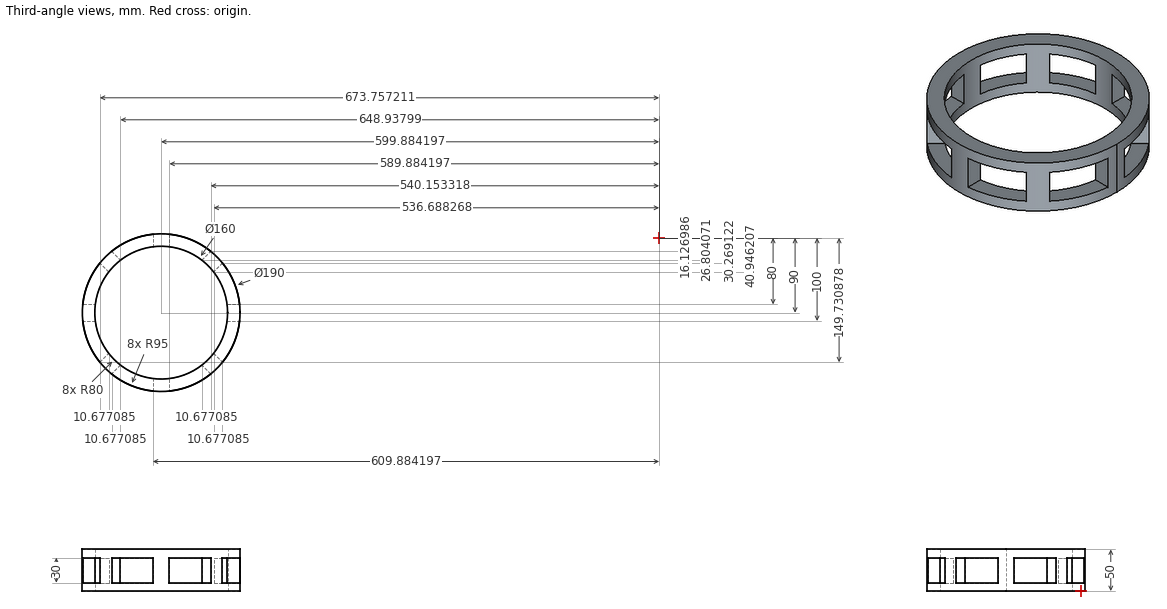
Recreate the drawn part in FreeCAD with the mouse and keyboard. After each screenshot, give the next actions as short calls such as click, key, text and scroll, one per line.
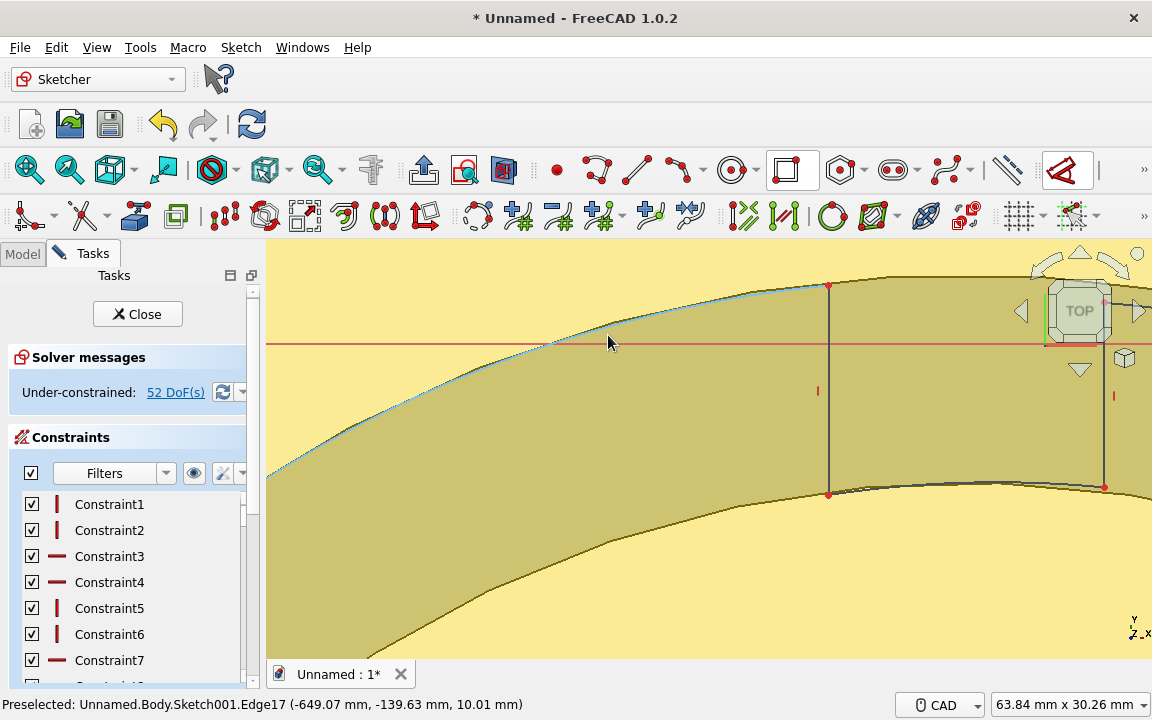
click(606, 327)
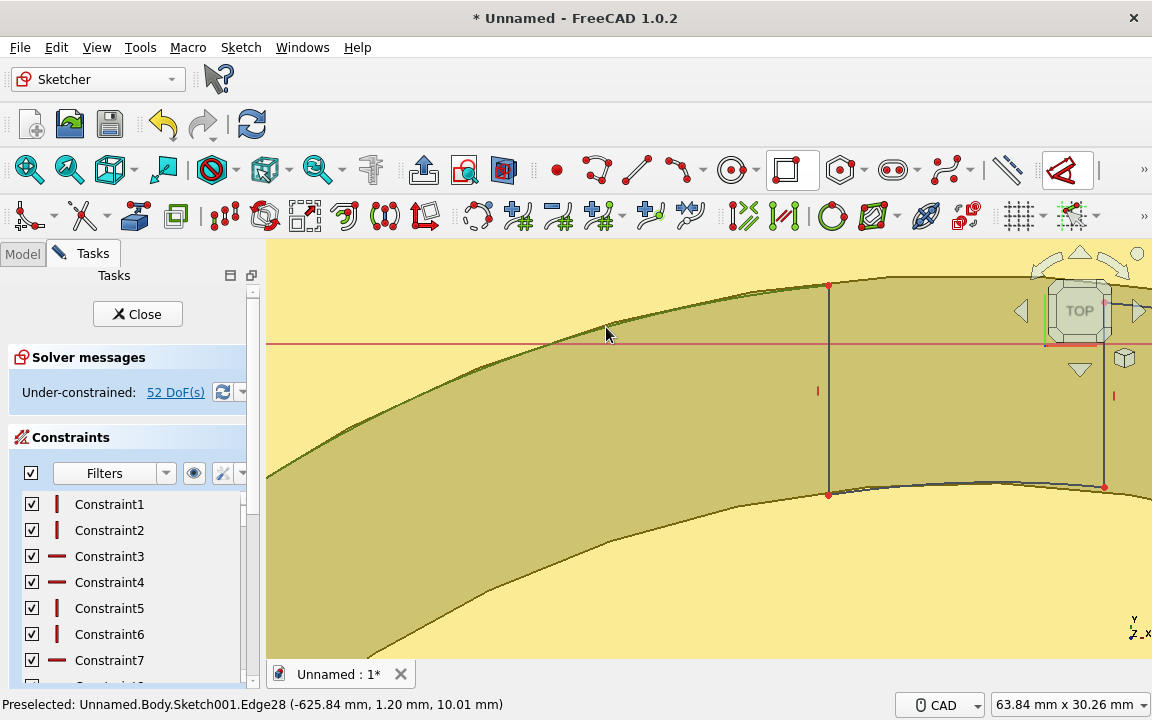
key(c)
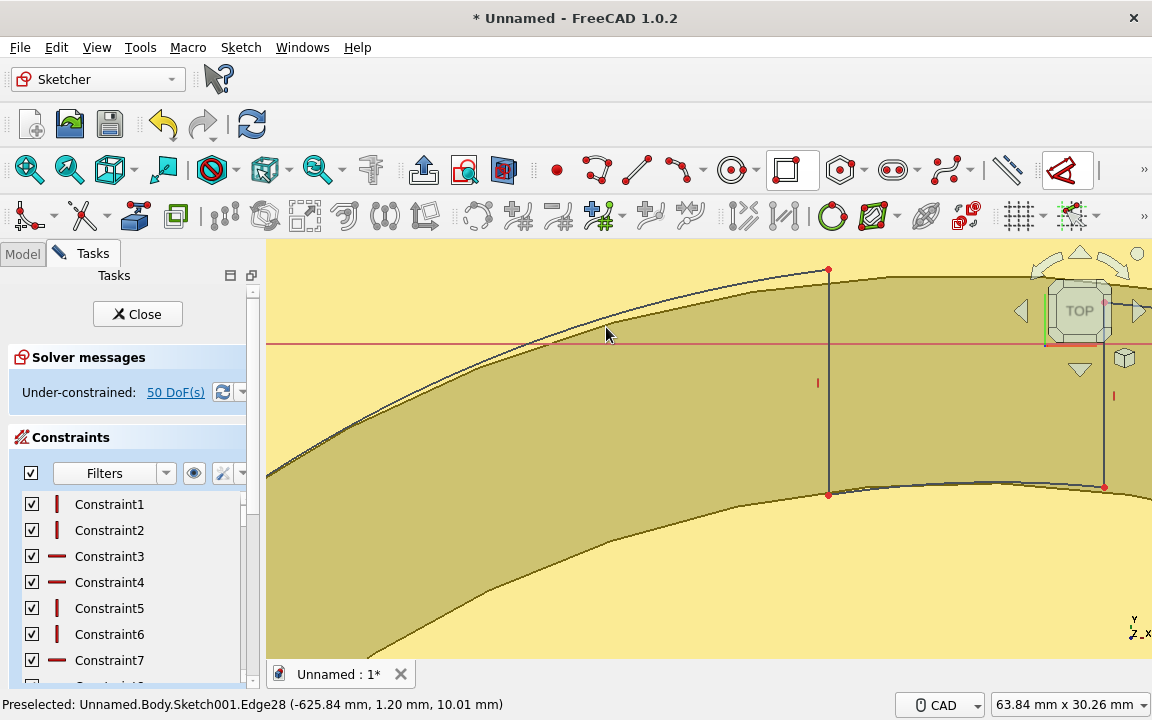
scroll(608, 335, down, 12)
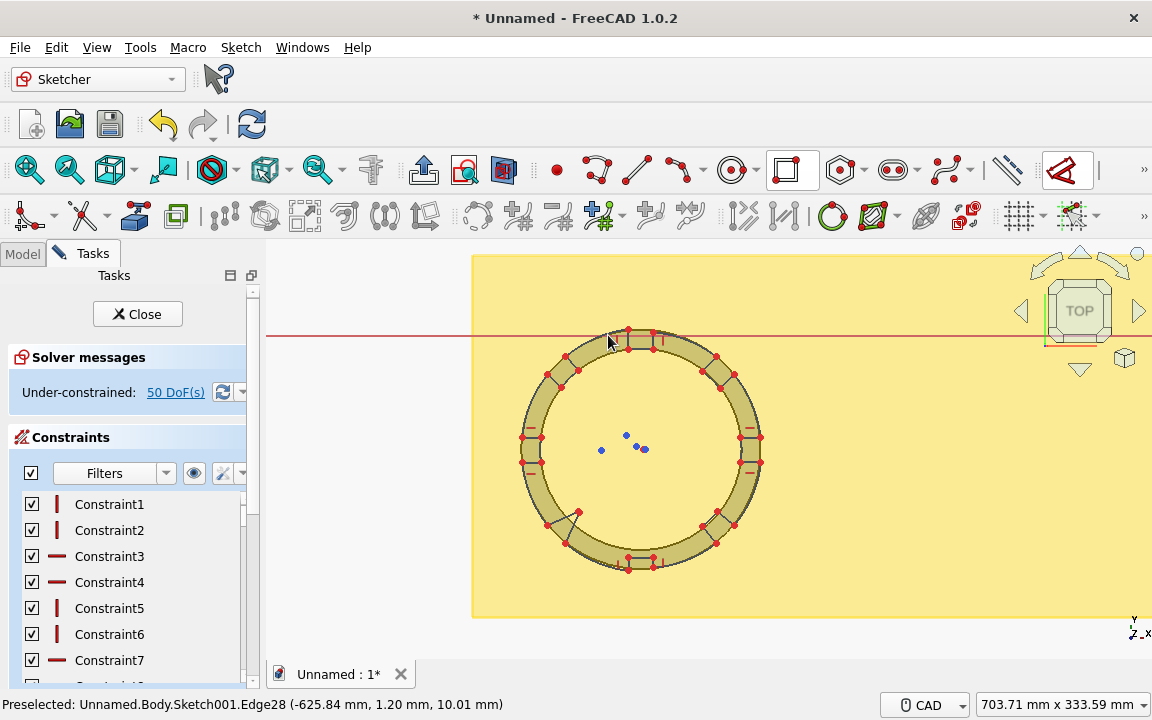
scroll(579, 512, up, 15)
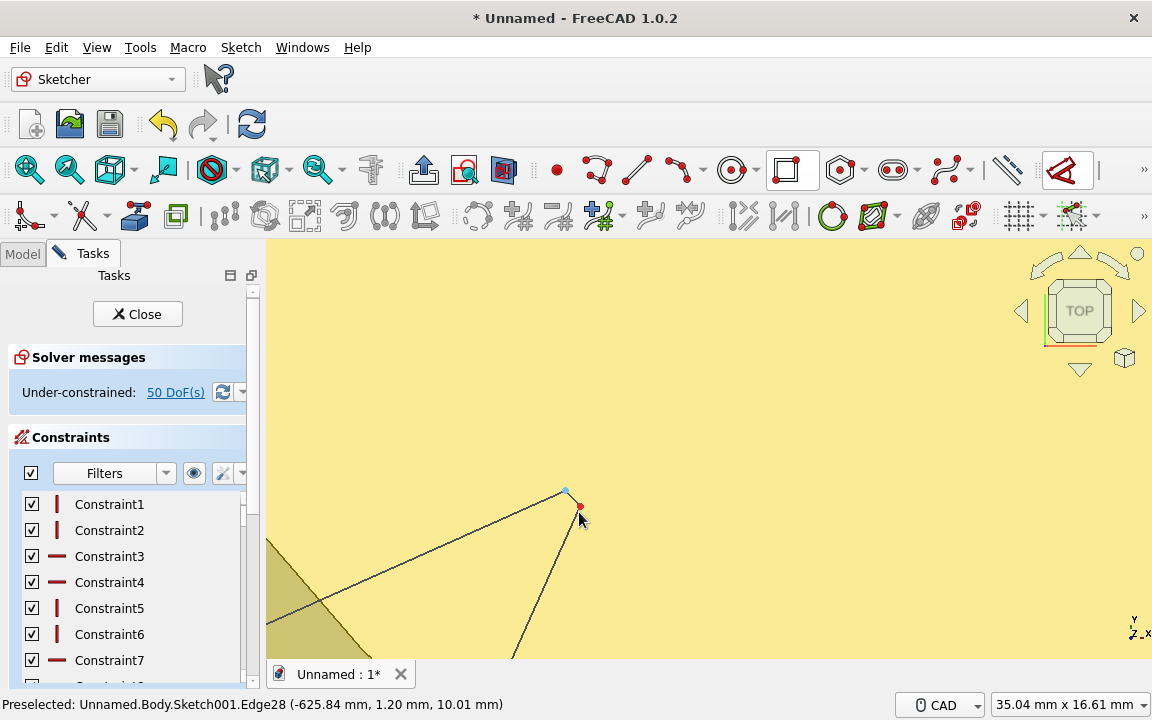
click(573, 499)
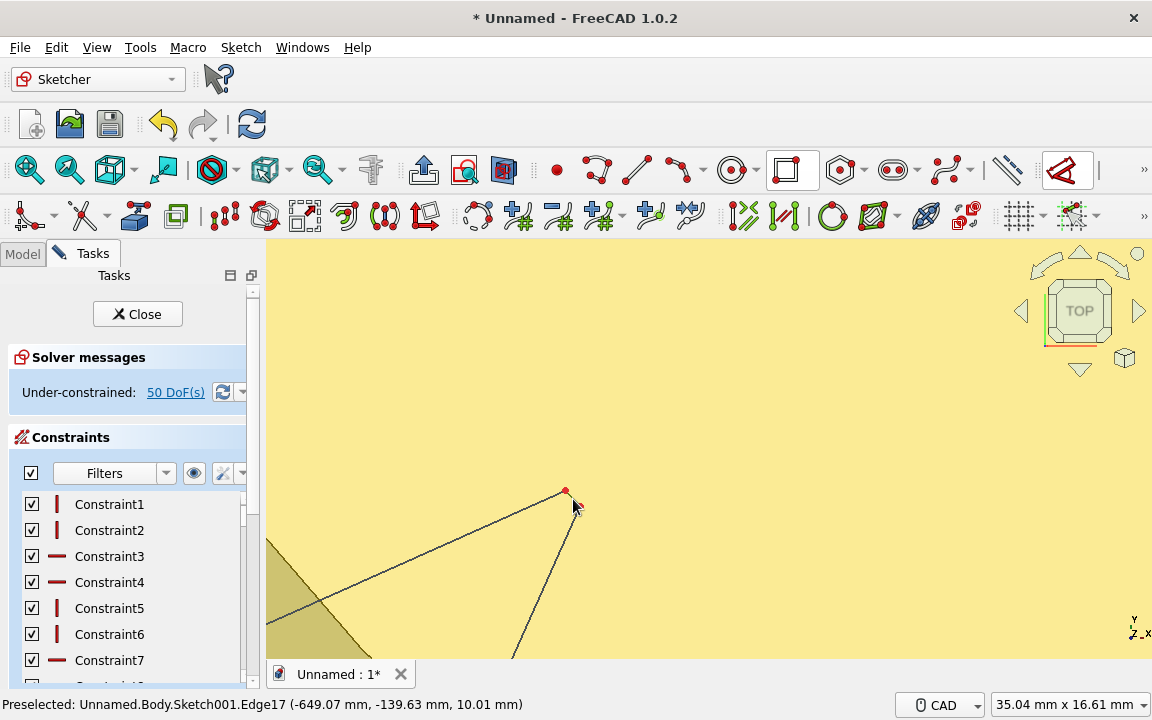
scroll(579, 512, down, 15)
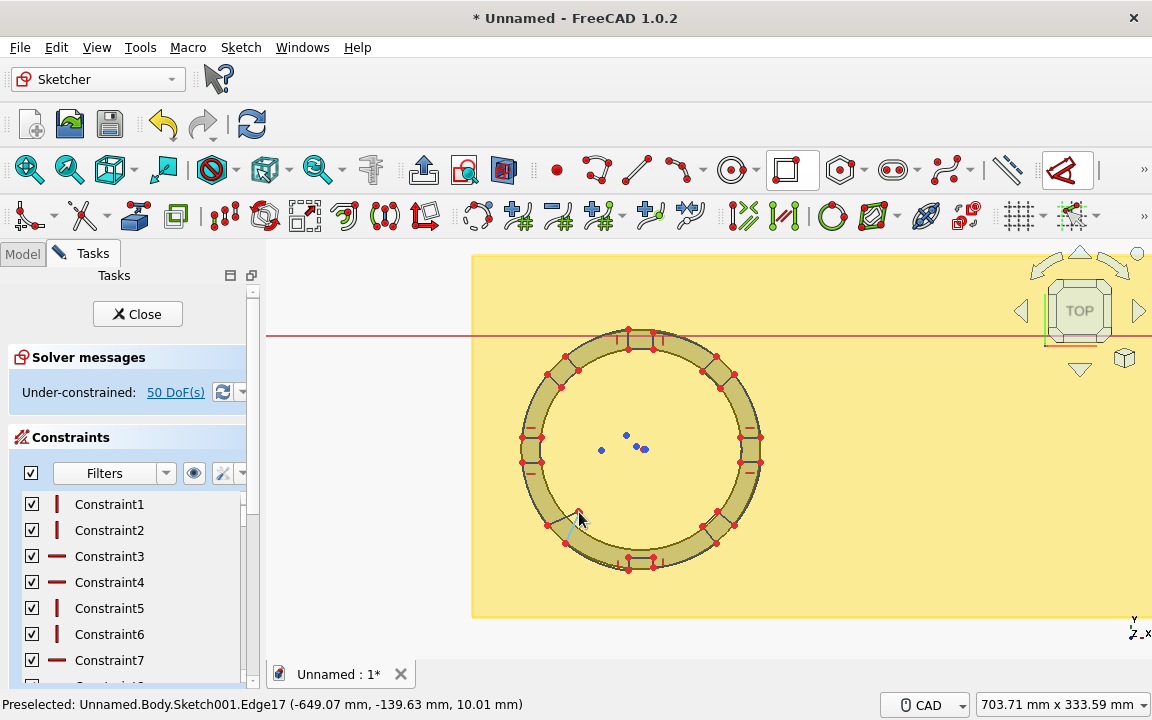
scroll(573, 375, up, 4)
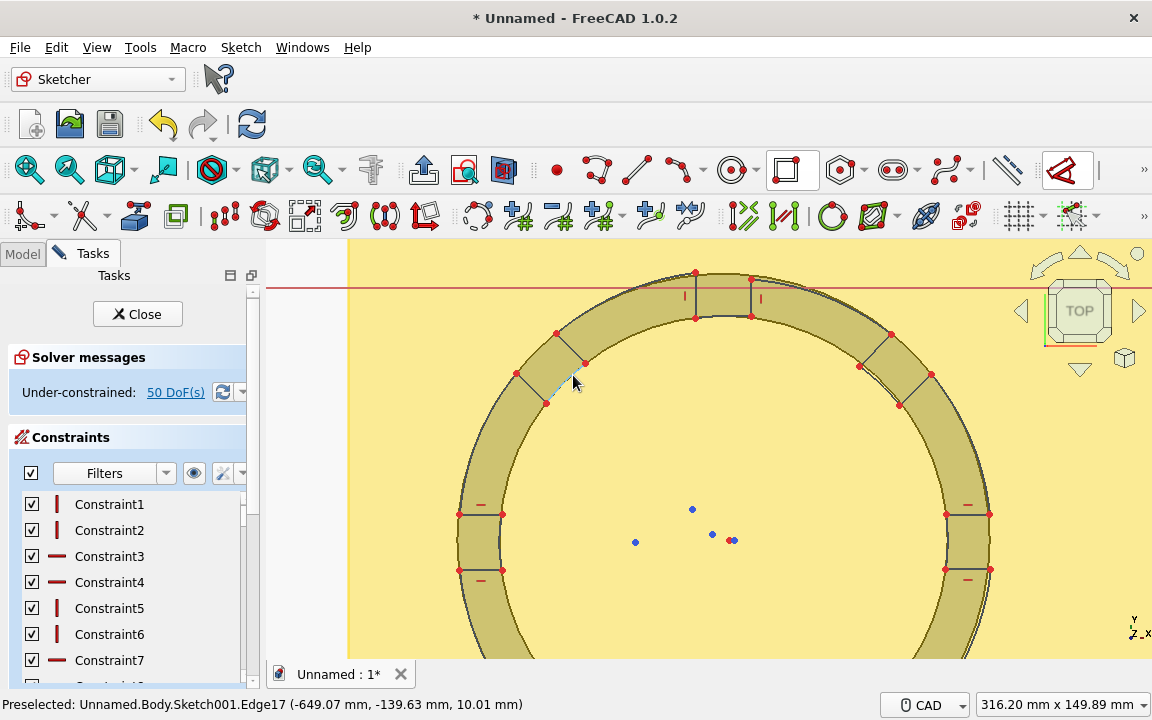
click(573, 374)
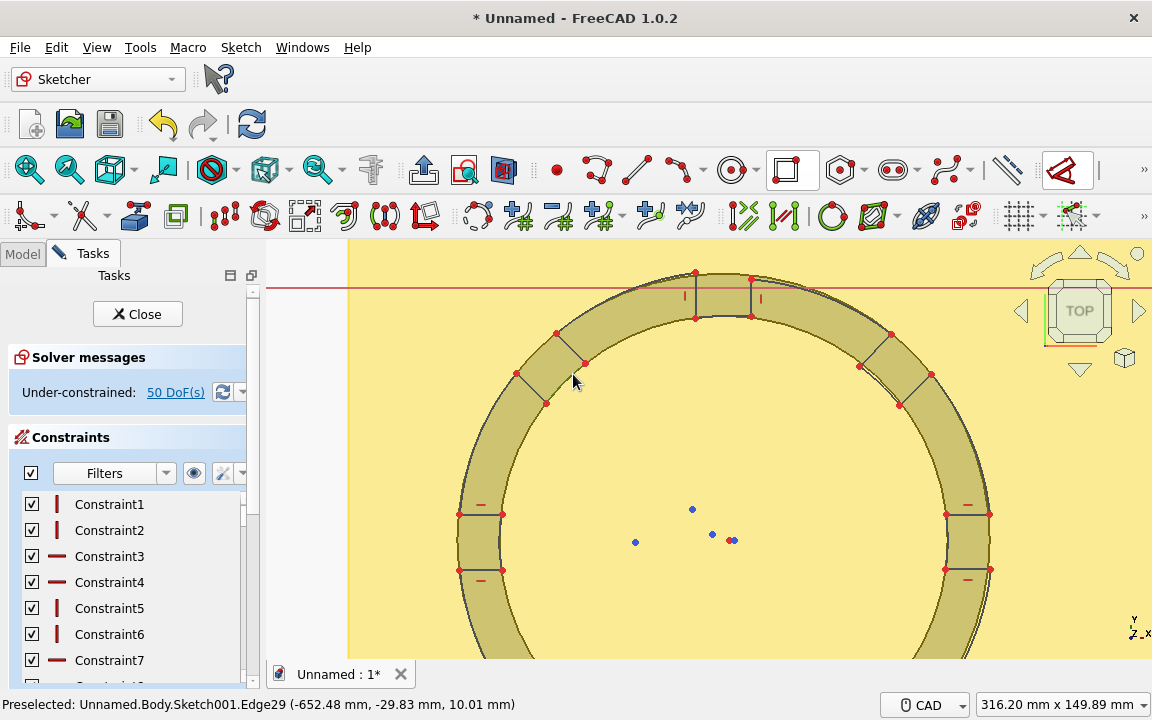
key(c)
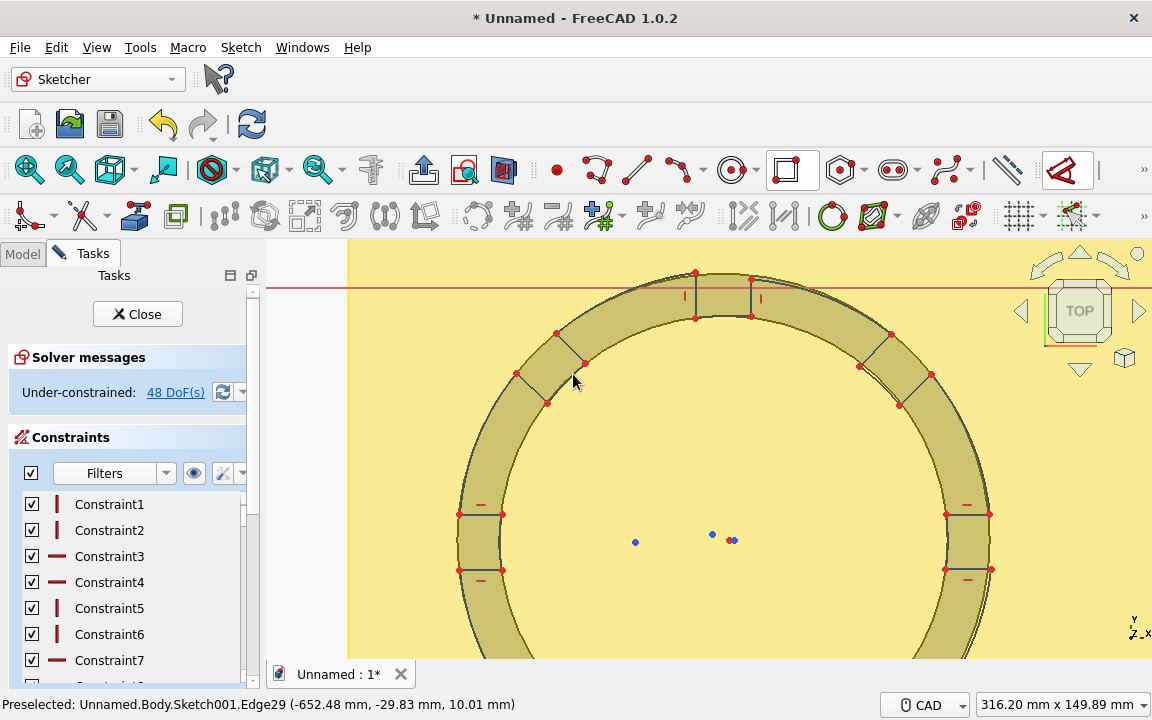
scroll(573, 375, down, 4)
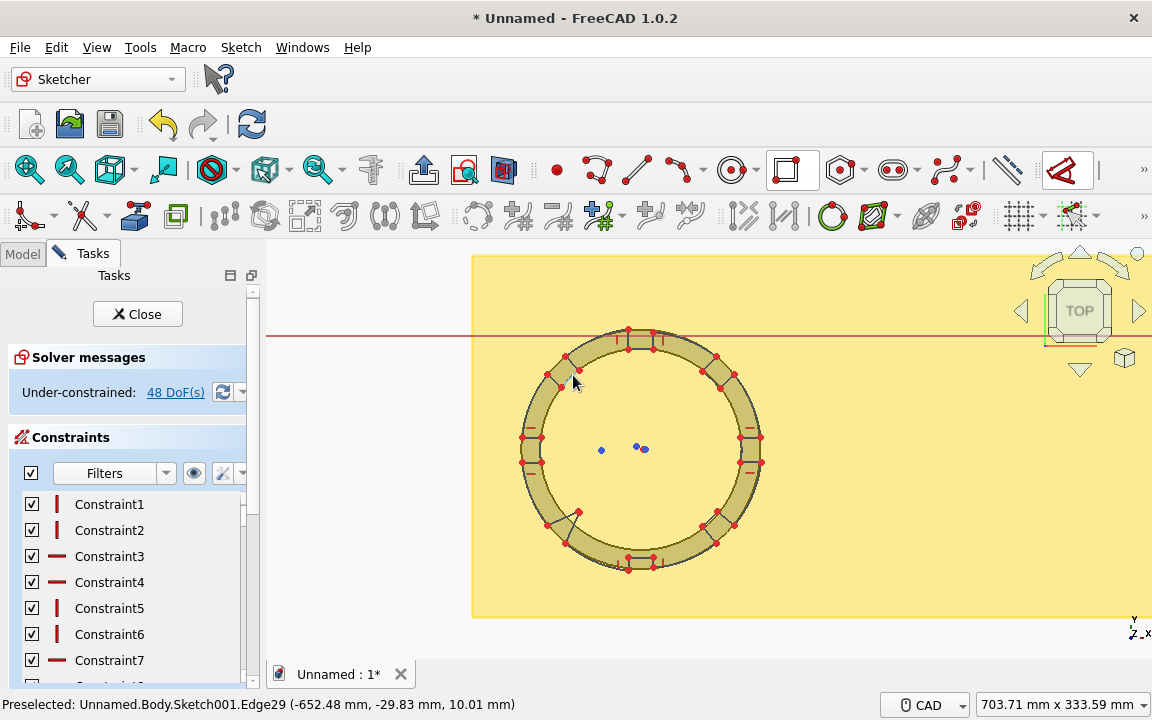
scroll(579, 512, up, 15)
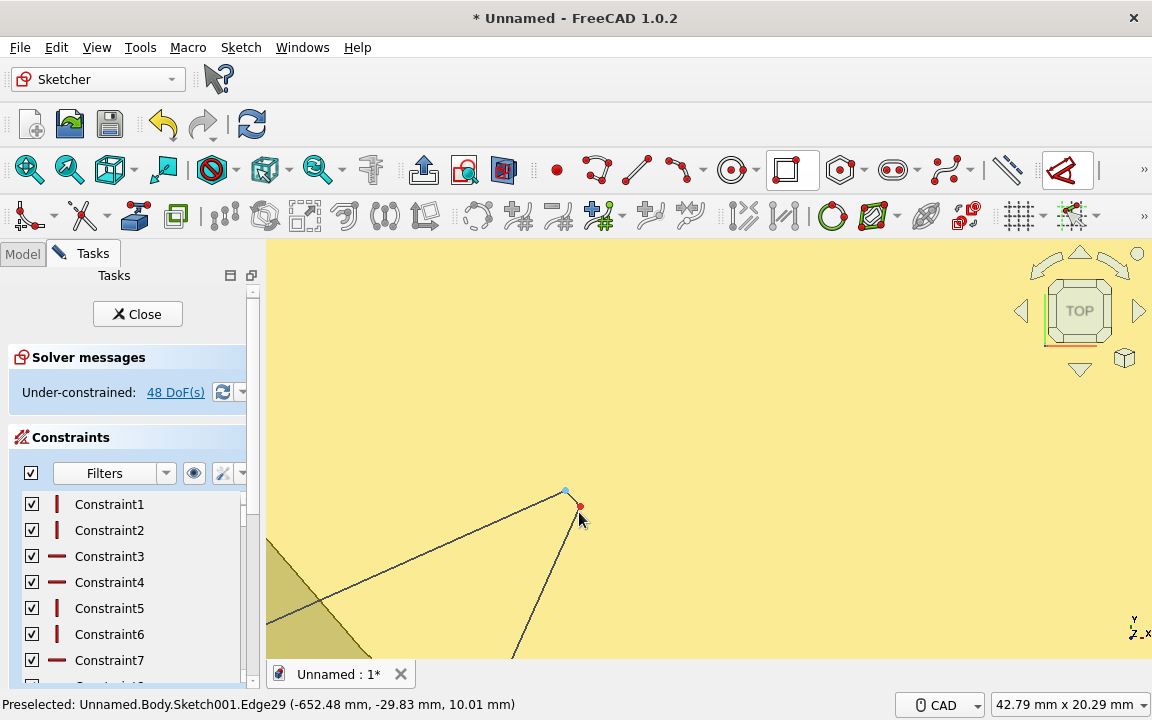
click(573, 499)